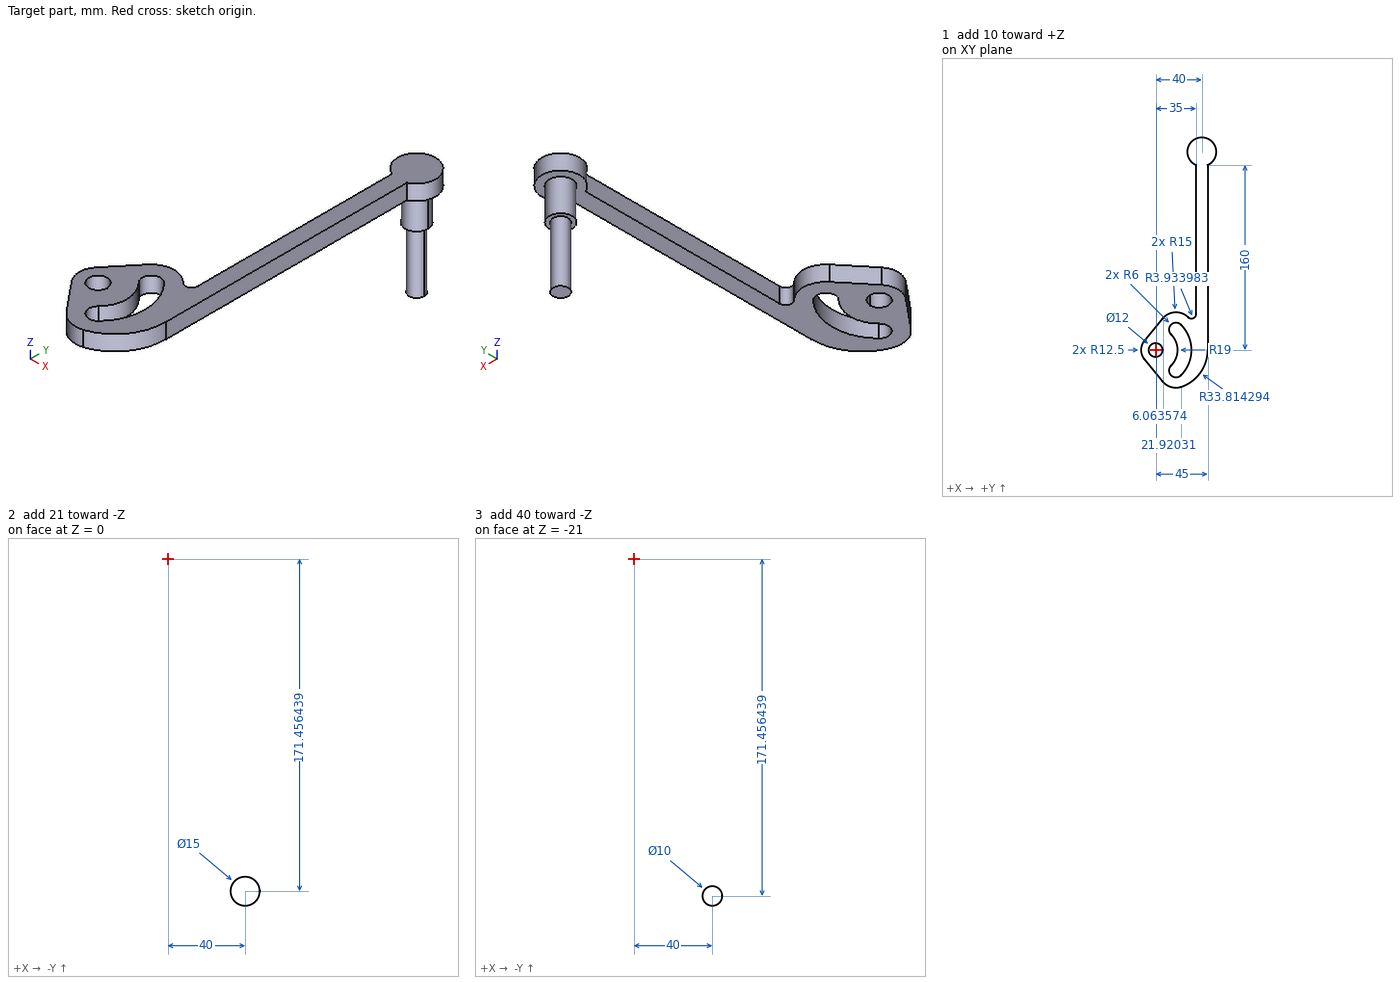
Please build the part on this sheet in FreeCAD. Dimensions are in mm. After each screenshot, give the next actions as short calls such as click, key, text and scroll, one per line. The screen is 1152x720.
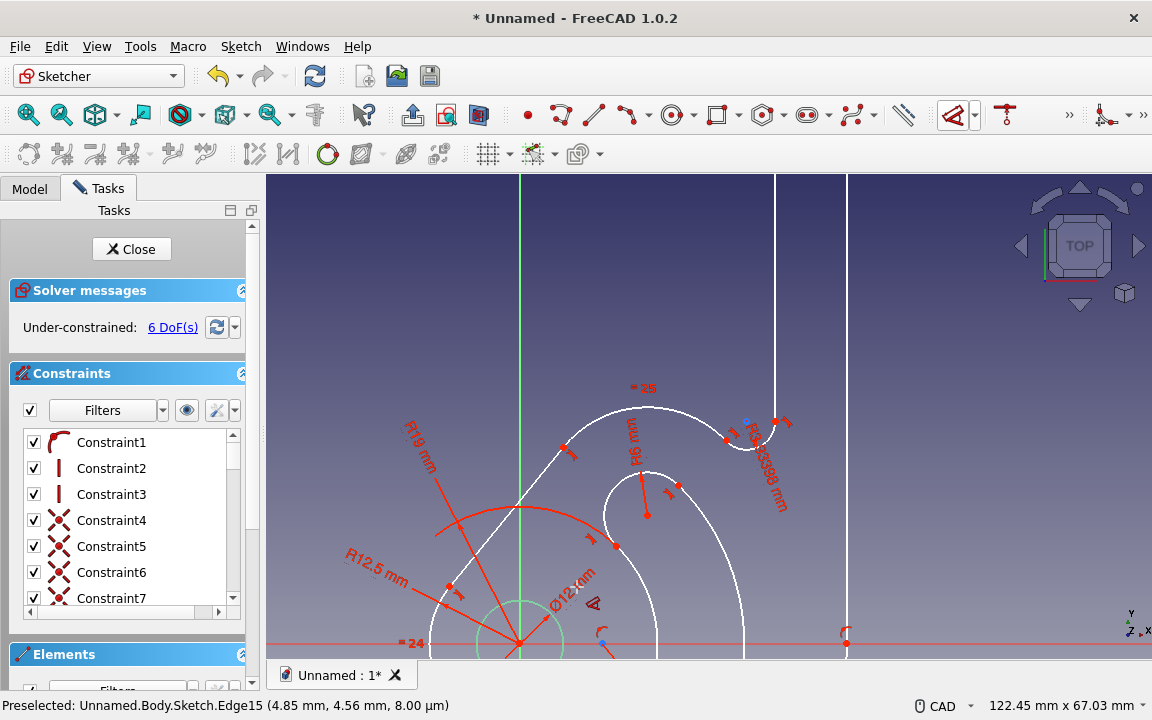
scroll(641, 498, down, 8)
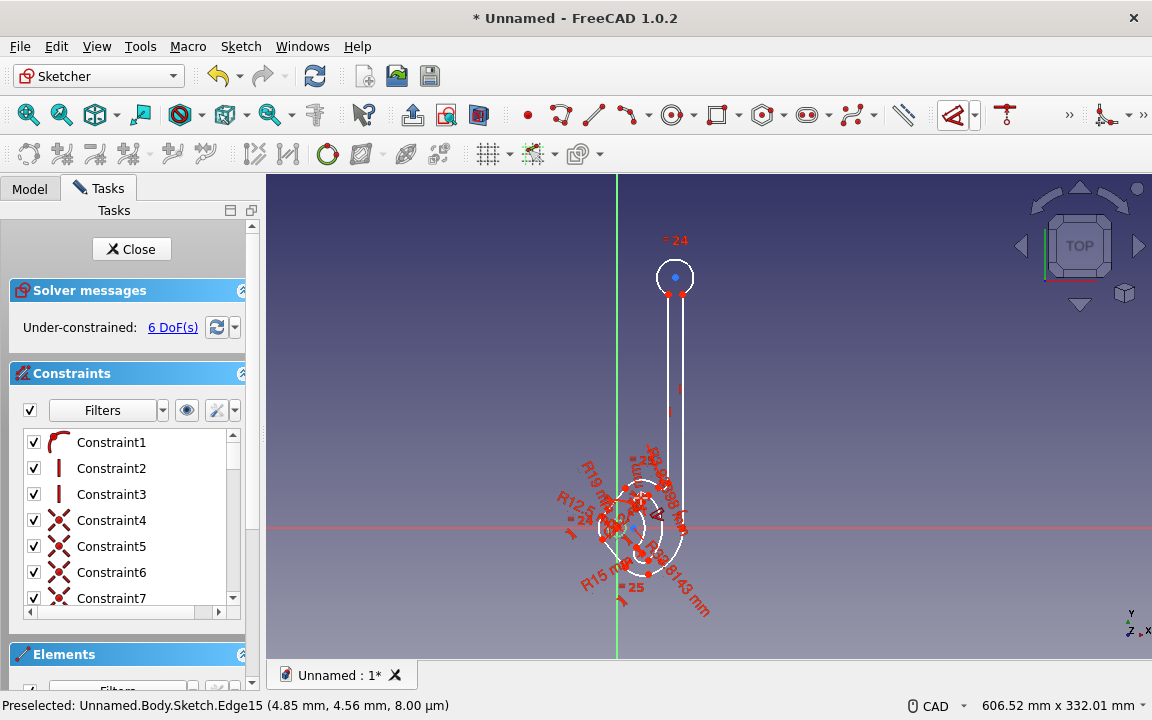
click(683, 458)
click(717, 411)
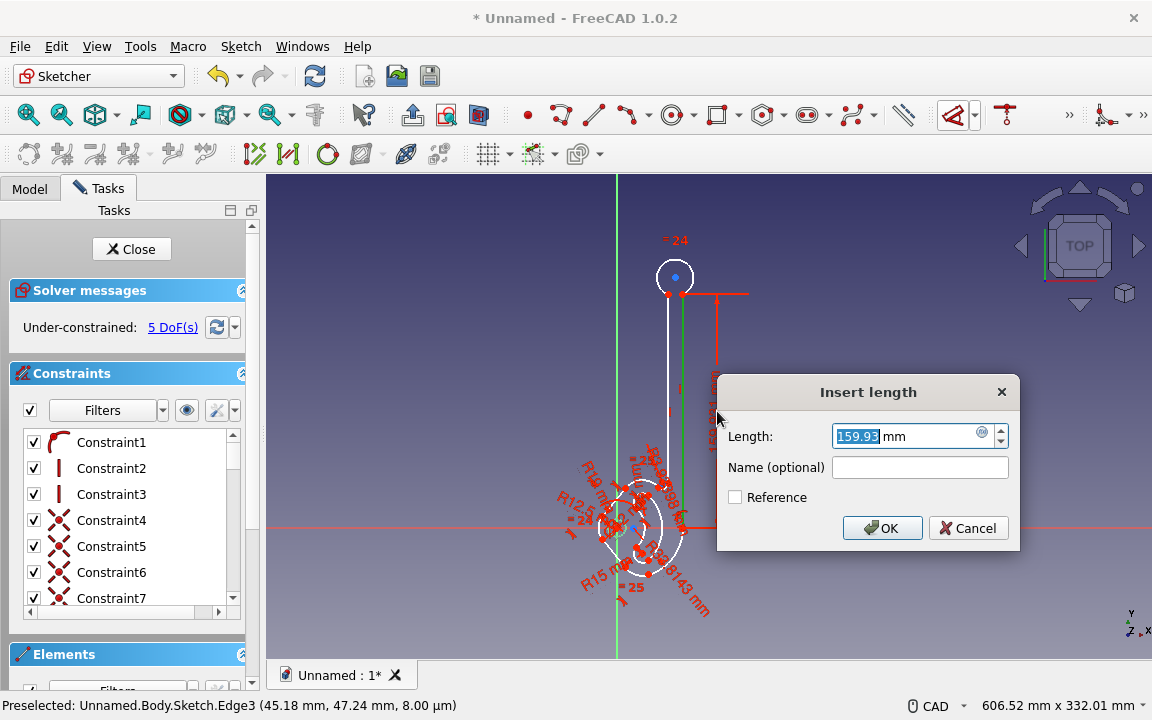
text(160)
key(Return)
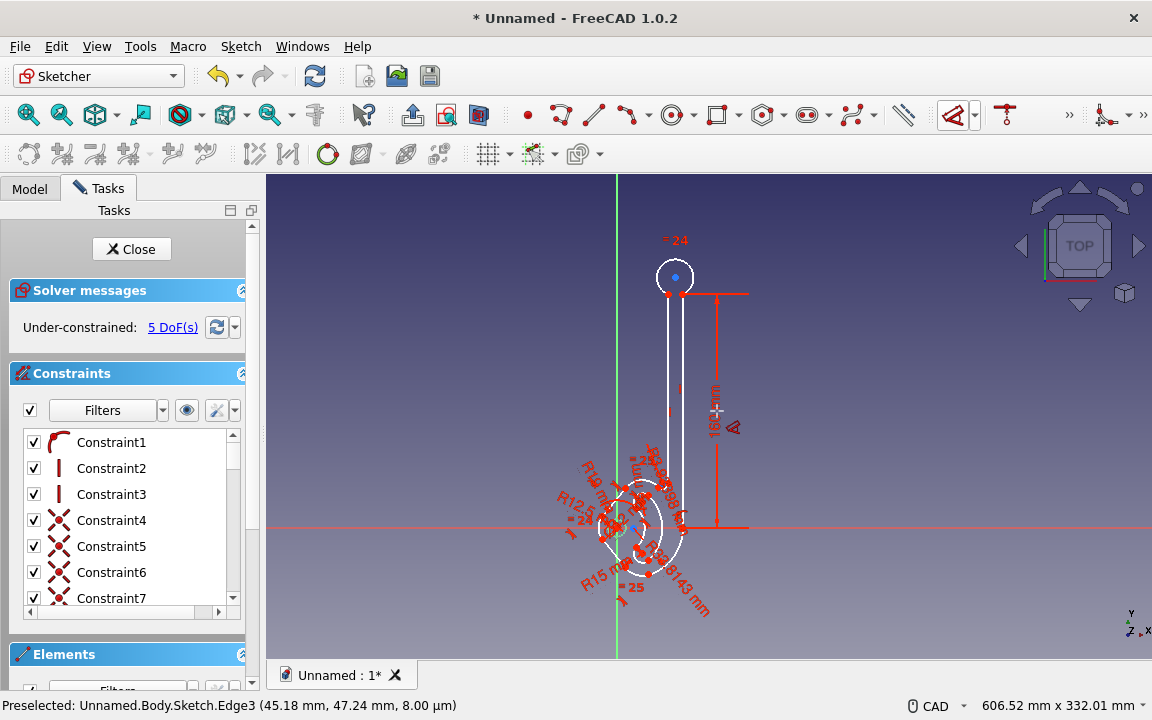
click(683, 528)
click(650, 610)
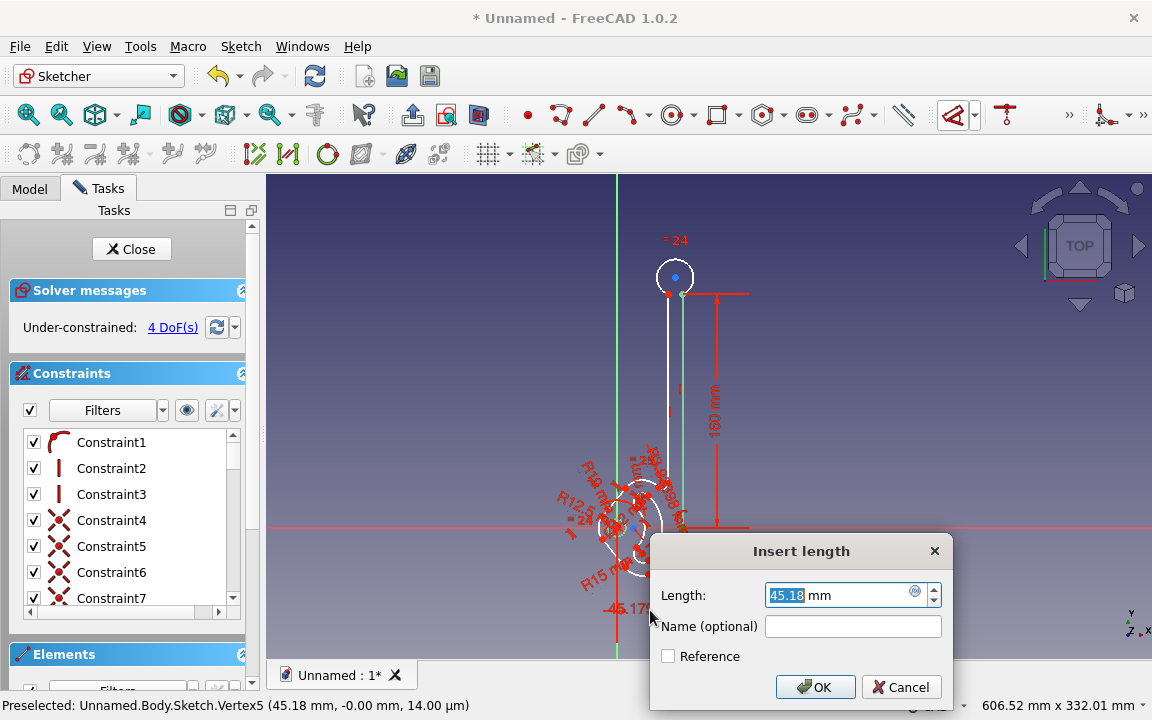
text(45)
key(Return)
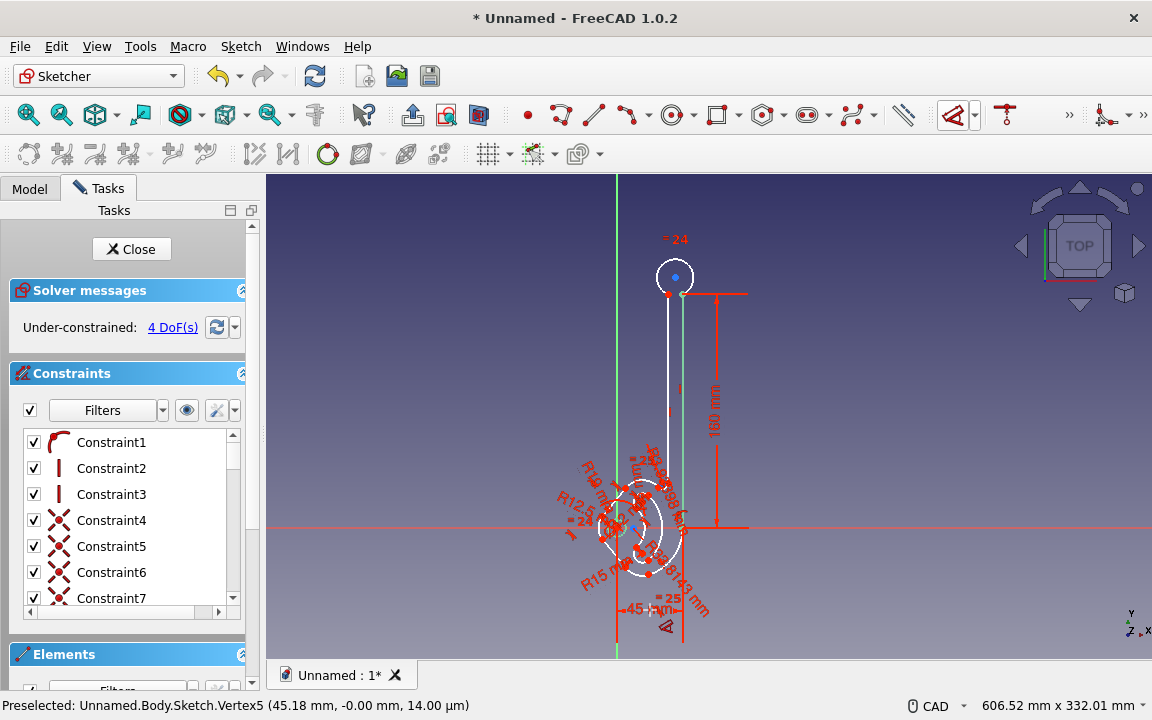
click(668, 295)
click(643, 261)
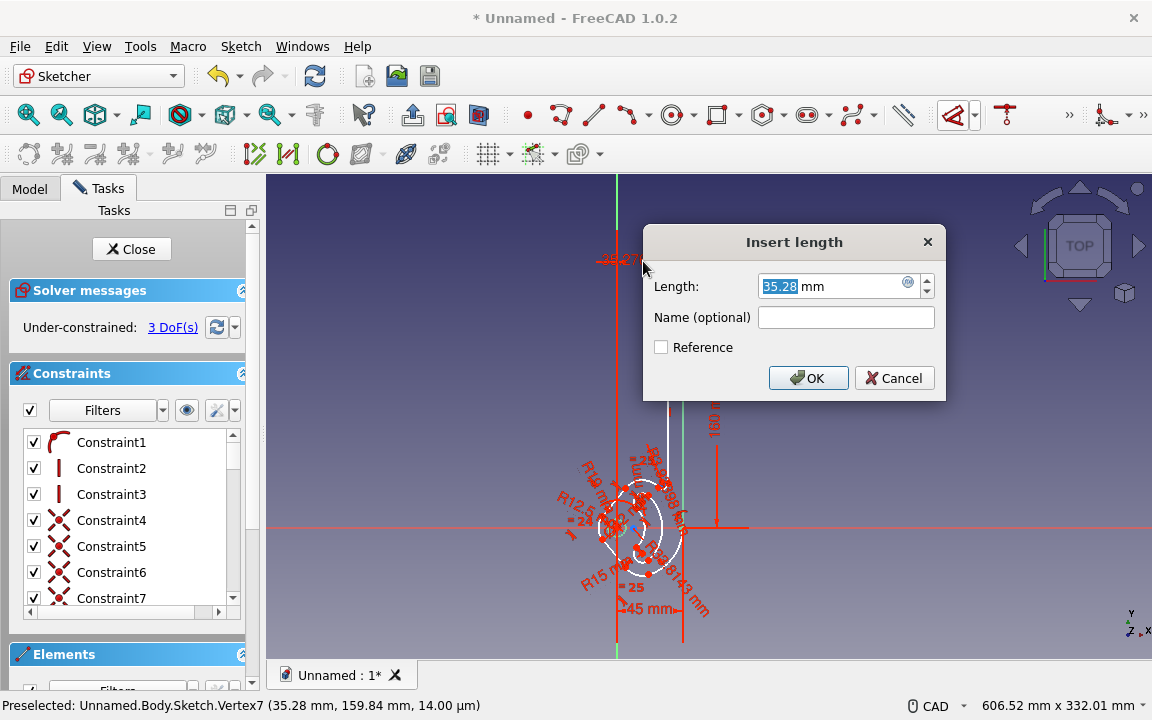
text(35)
key(Return)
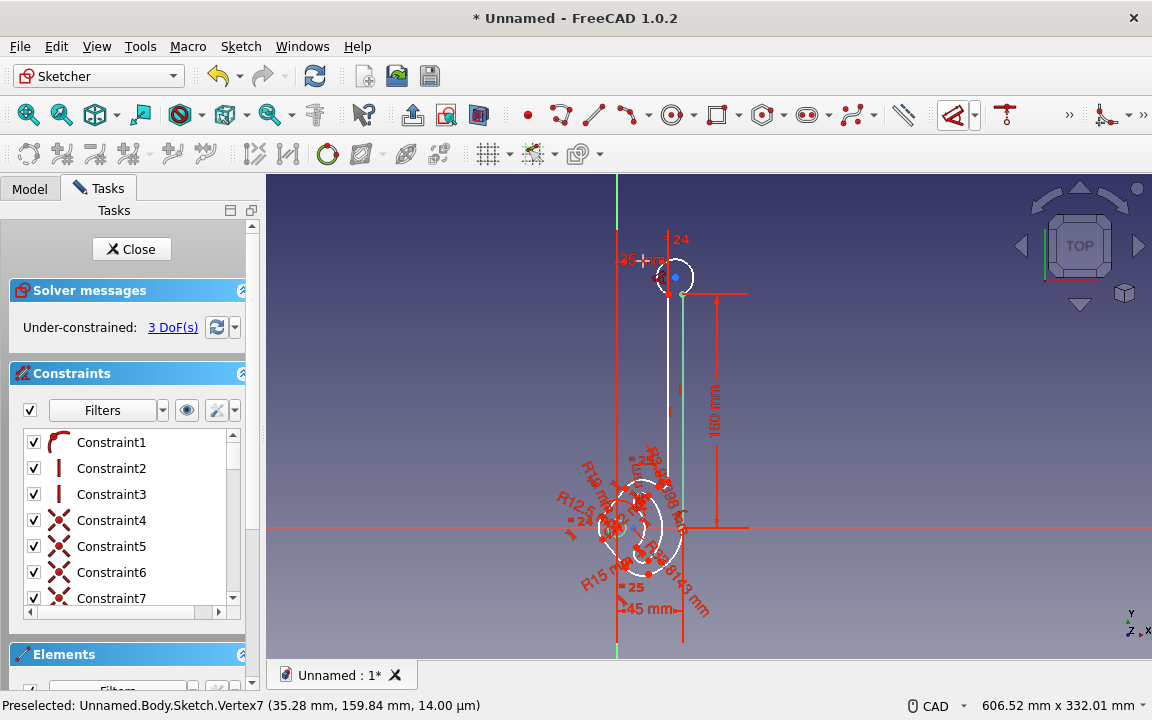
click(675, 278)
click(646, 220)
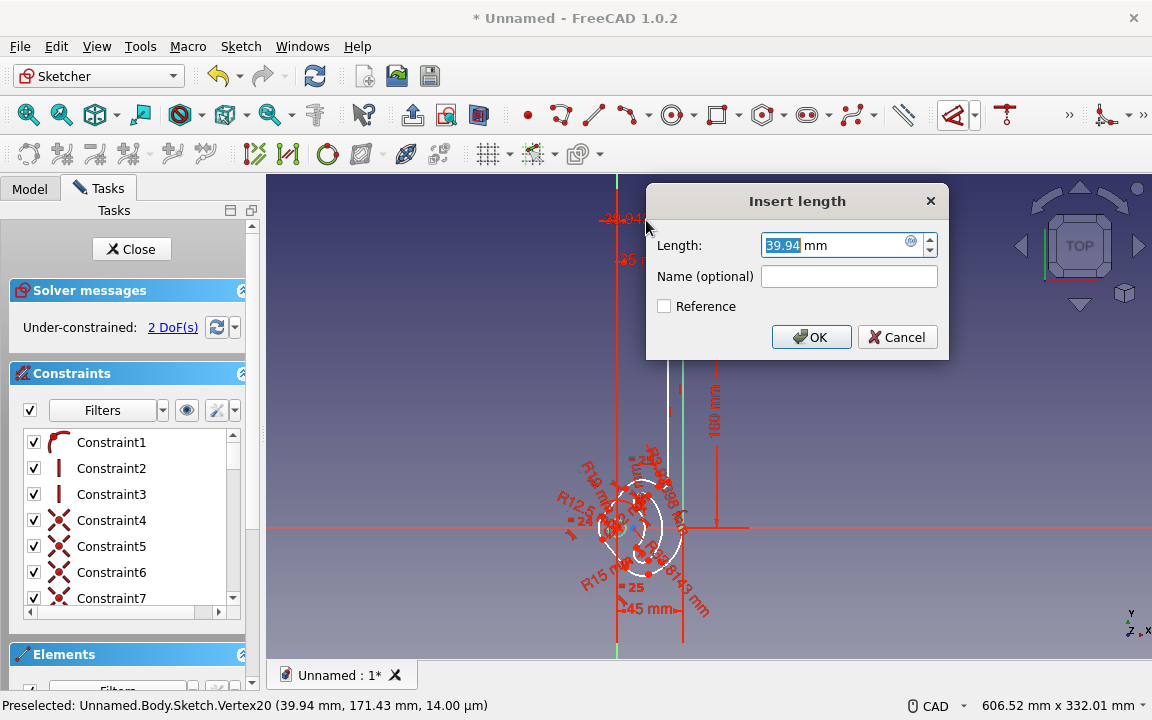
text(40)
key(Return)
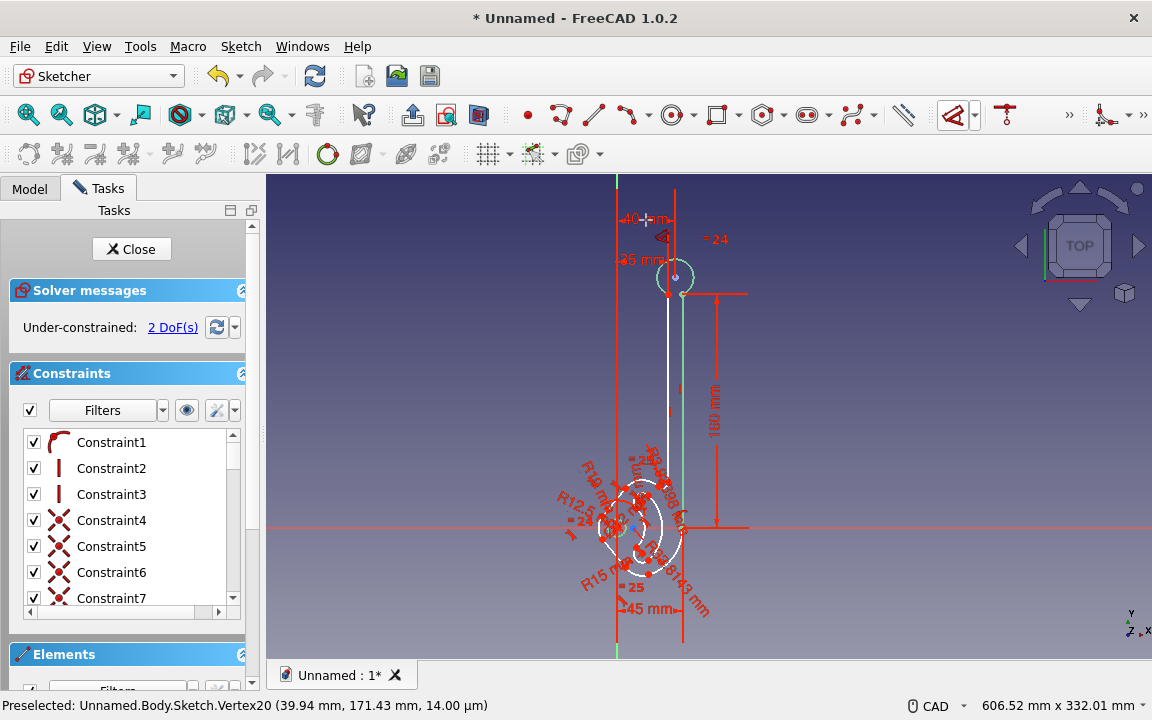
scroll(626, 488, up, 8)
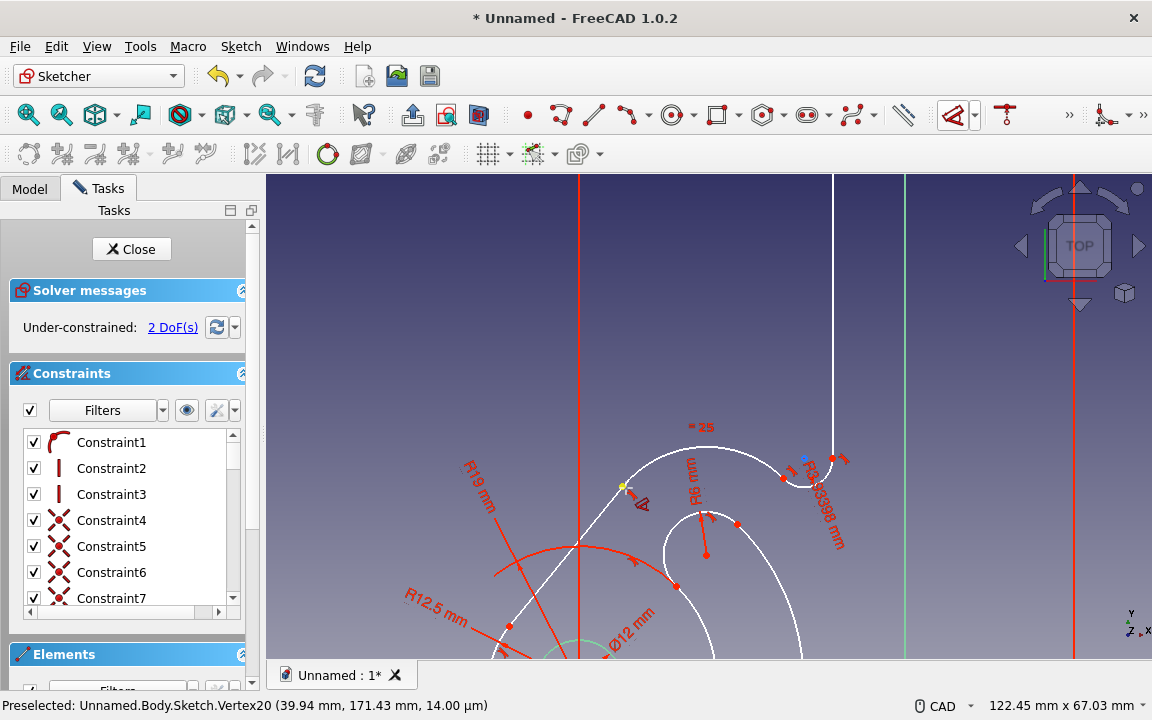
click(623, 487)
click(601, 453)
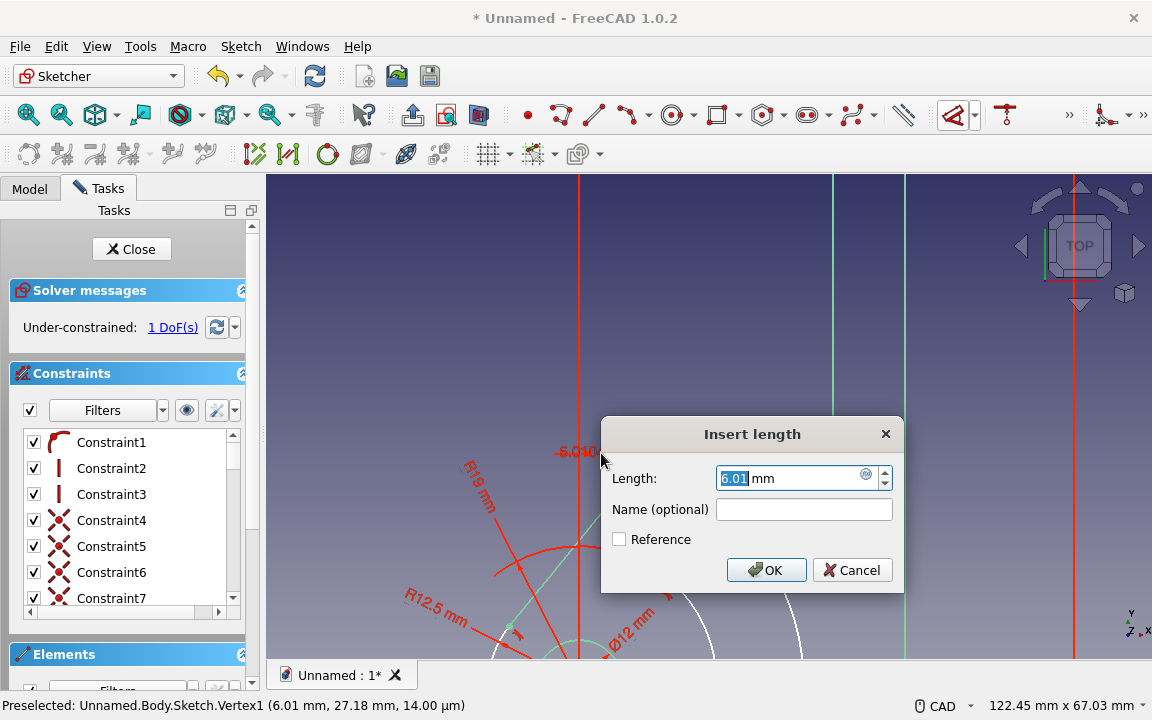
text(6.063574)
key(Return)